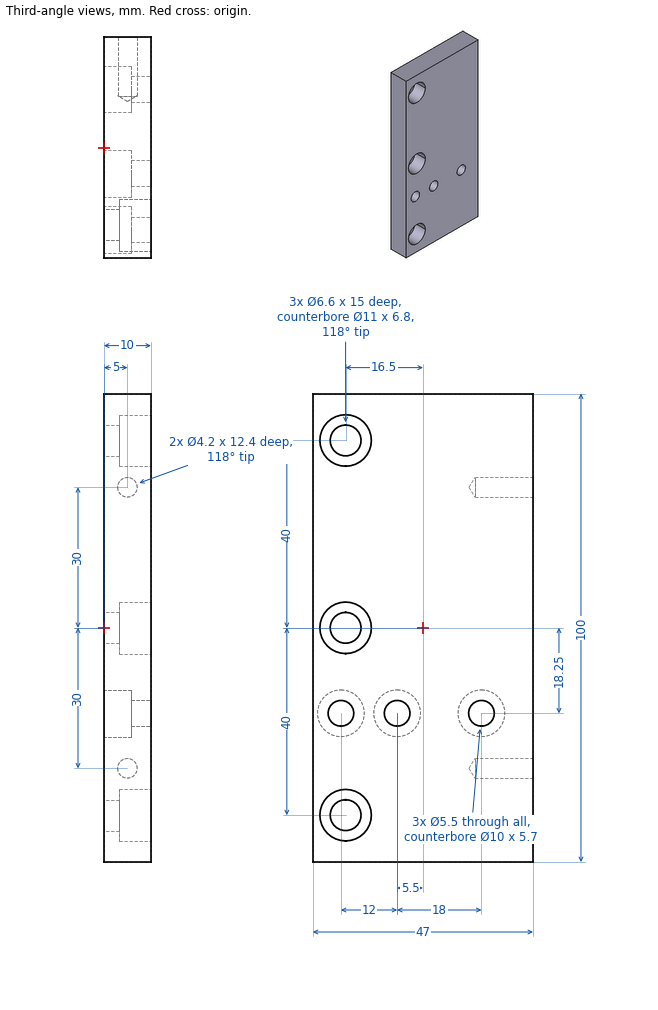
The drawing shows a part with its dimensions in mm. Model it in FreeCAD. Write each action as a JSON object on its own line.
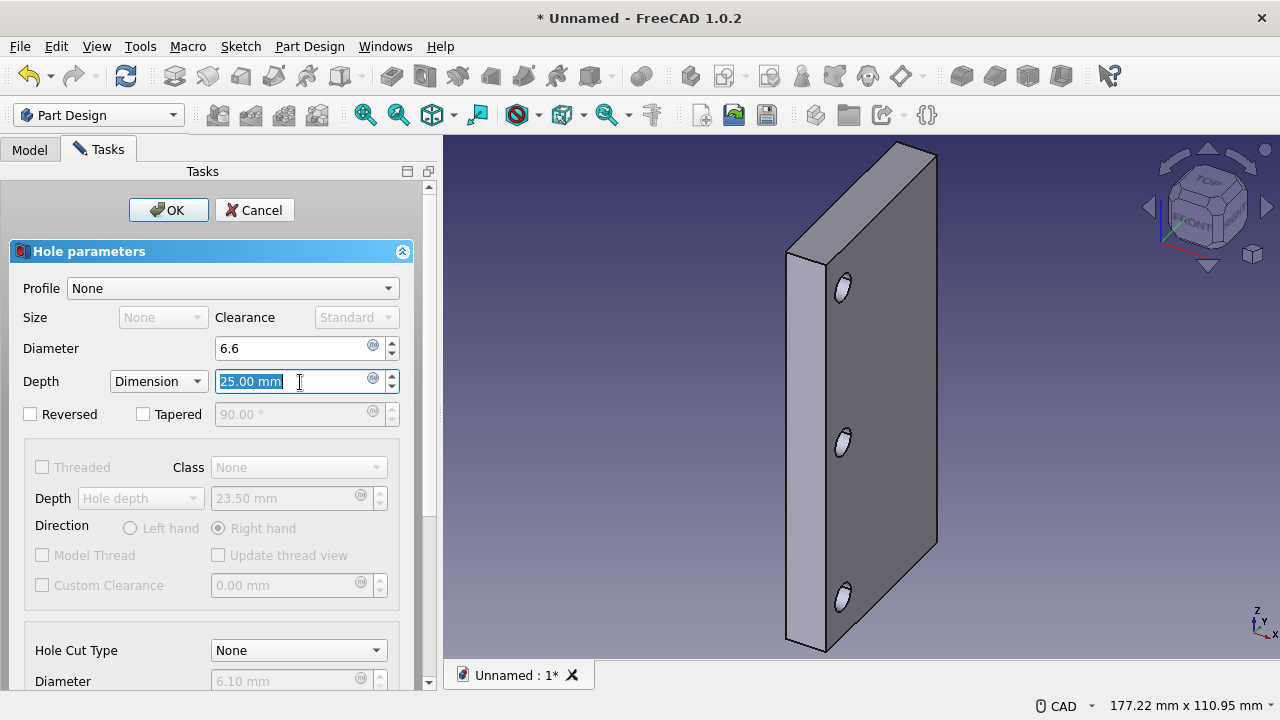
{"action": "type", "text": "15"}
{"action": "key", "text": "Tab"}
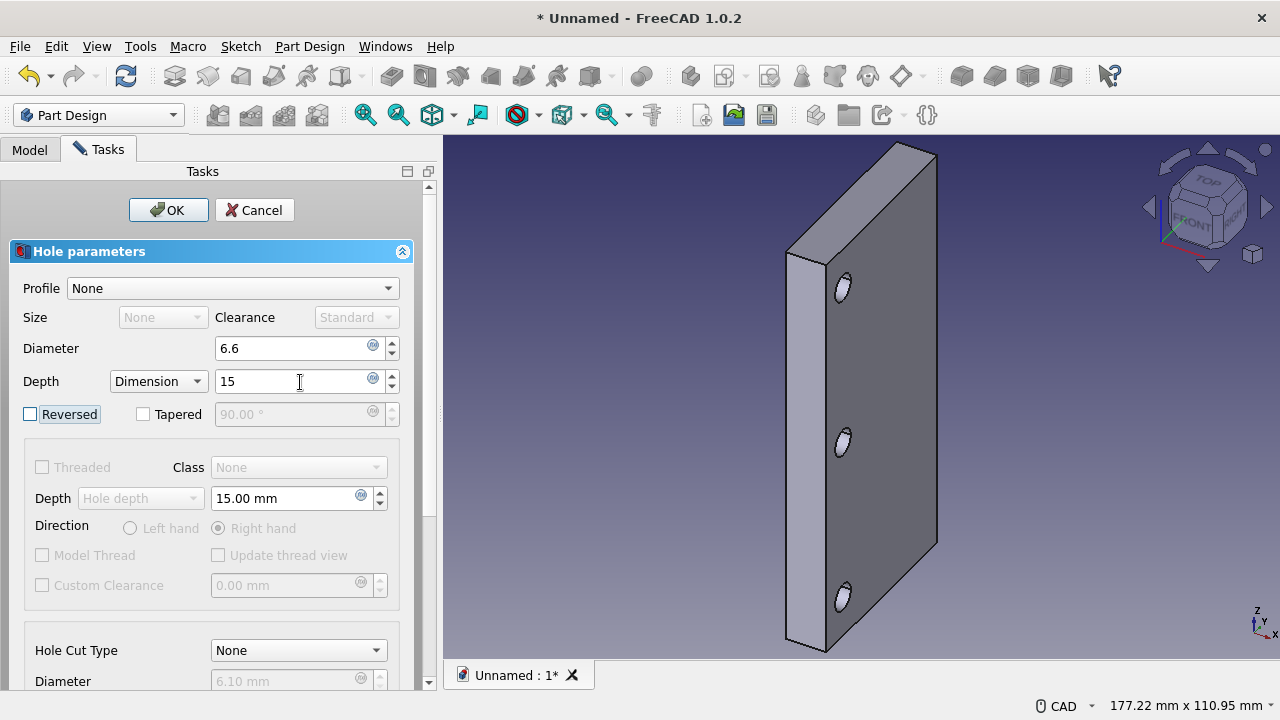
{"action": "left_click", "coordinate": [300, 650]}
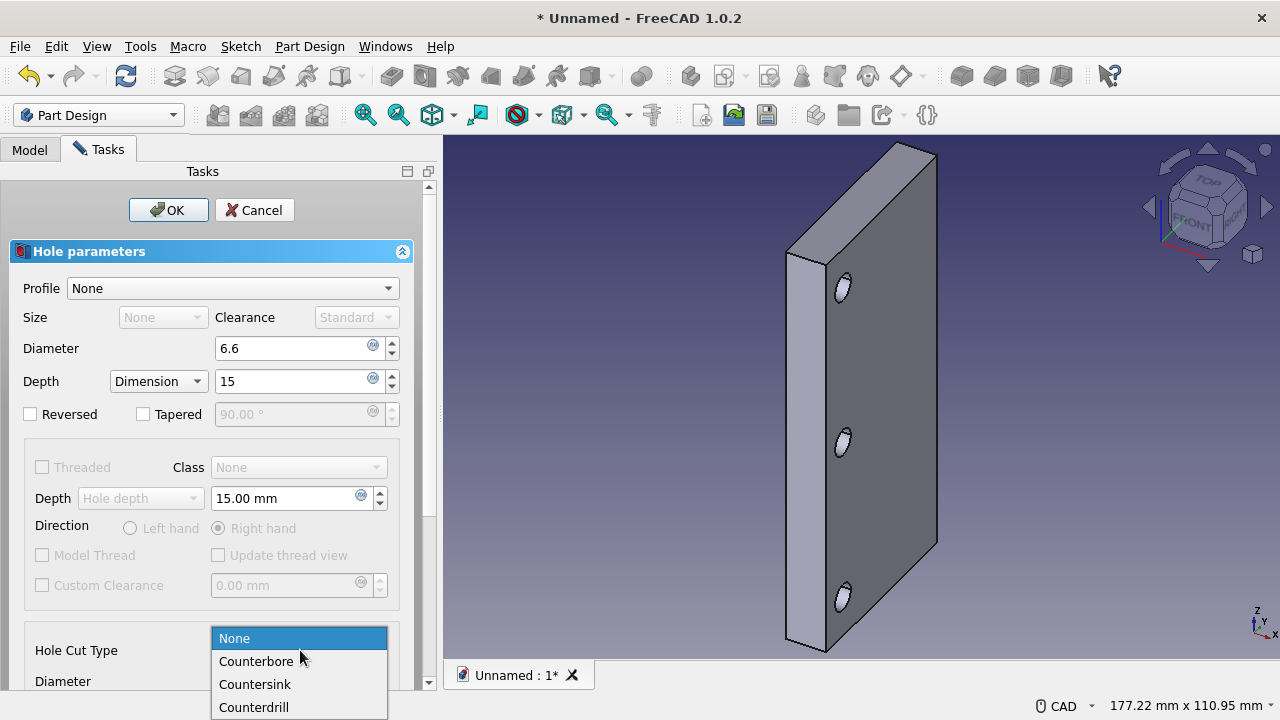
{"action": "left_click", "coordinate": [298, 662]}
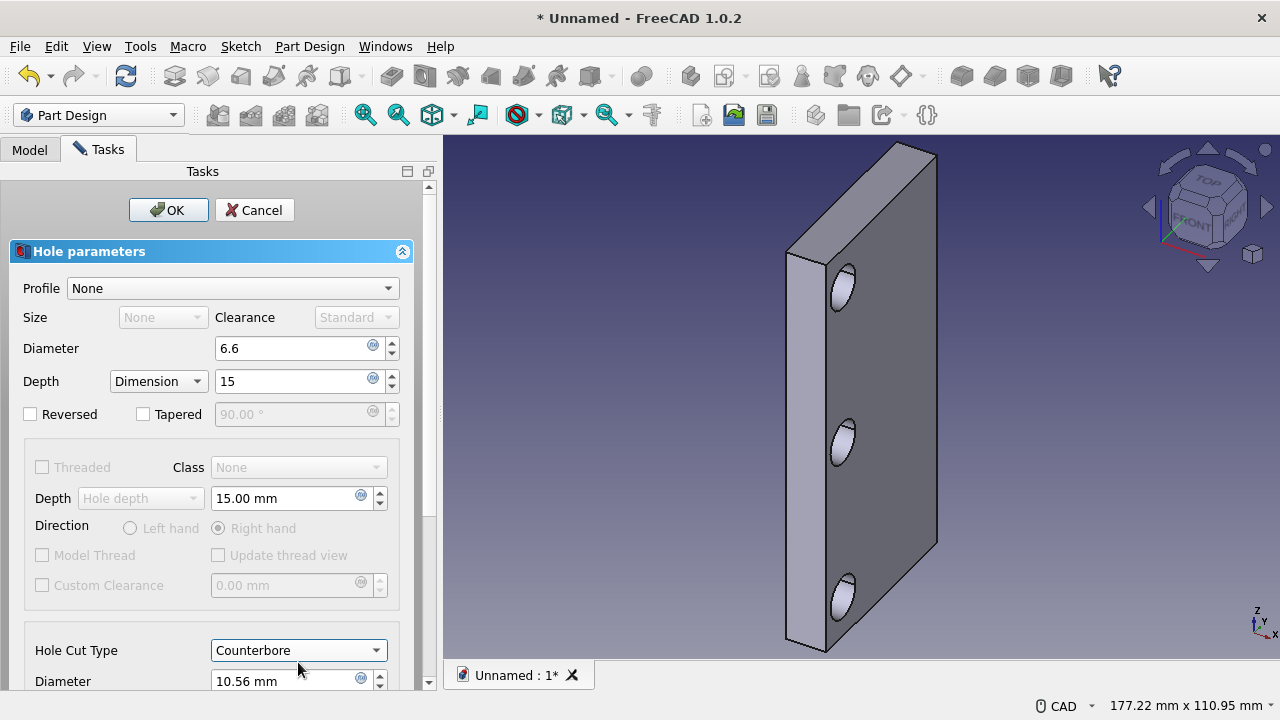
{"action": "scroll", "coordinate": [429, 436], "scroll_direction": "down", "scroll_amount": 2}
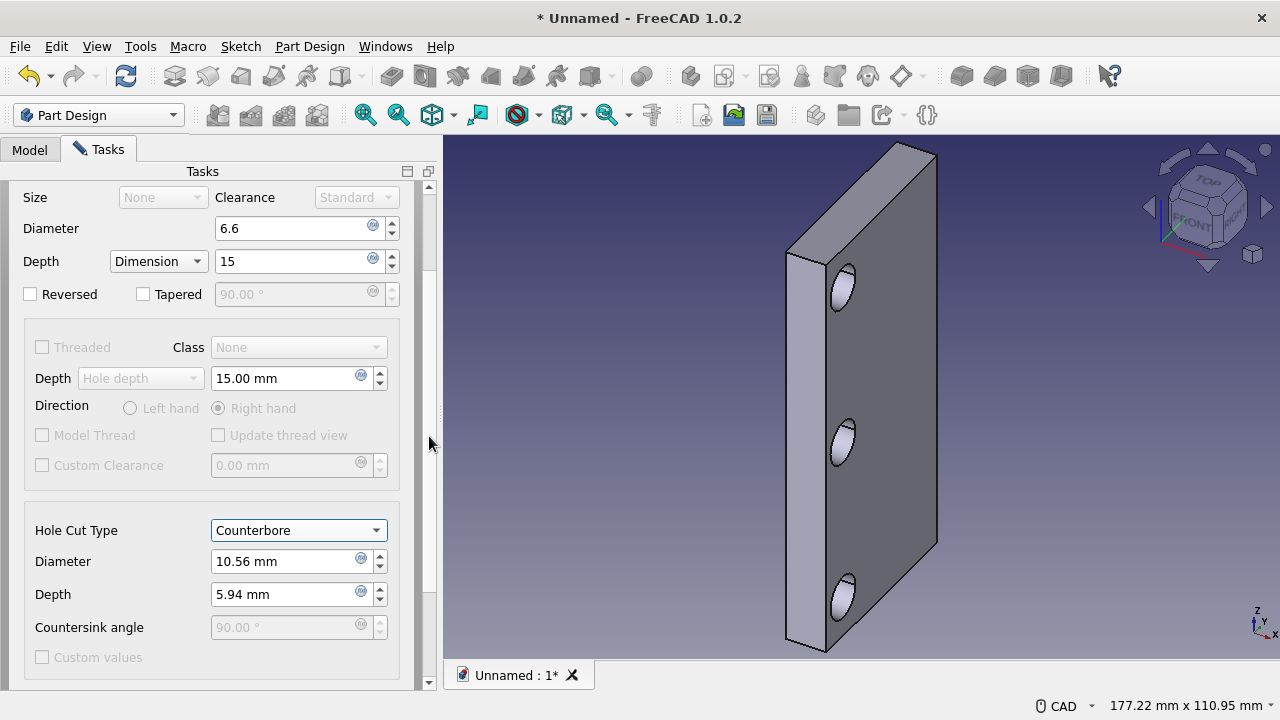
{"action": "triple_click", "coordinate": [292, 562]}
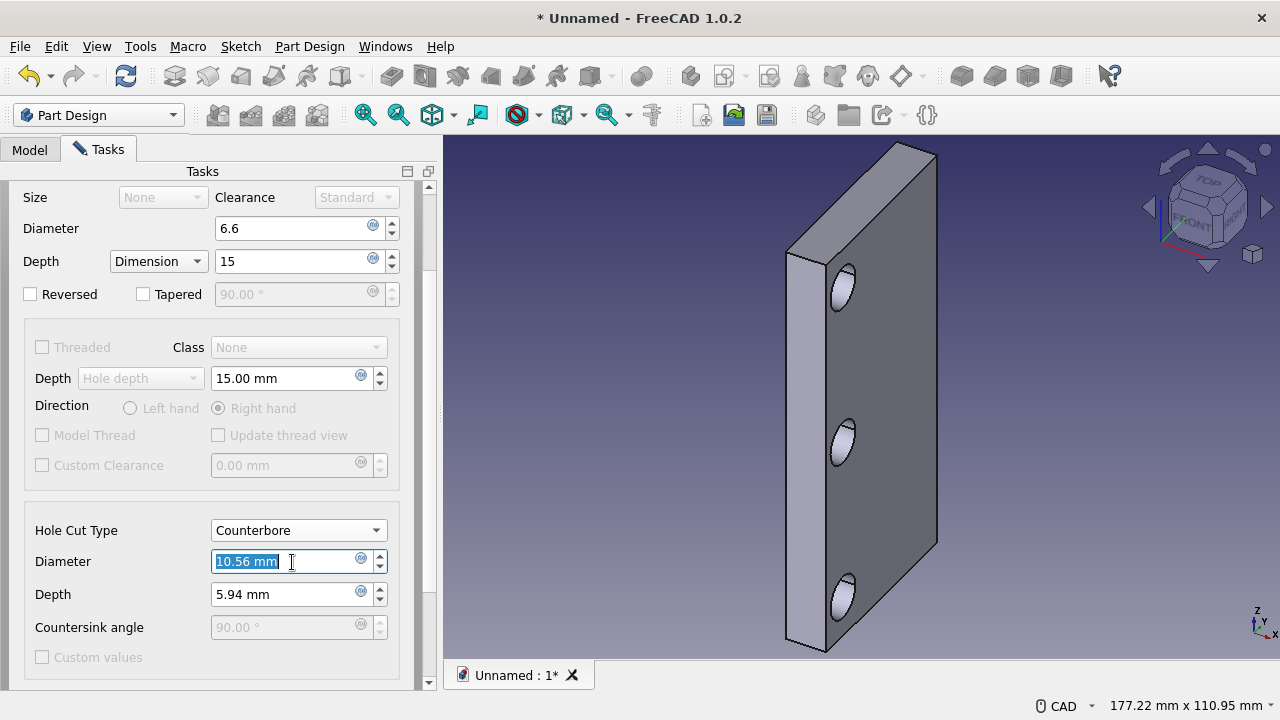
{"action": "type", "text": "11"}
{"action": "key", "text": "Tab"}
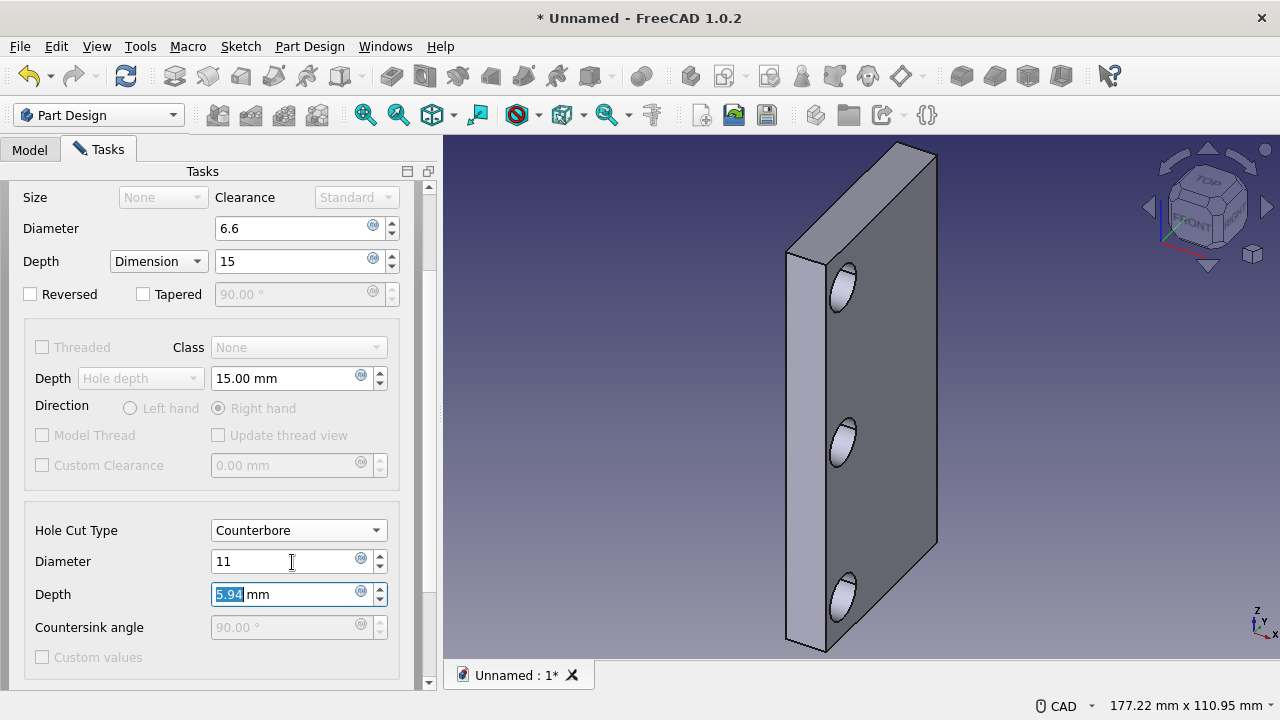
{"action": "type", "text": "6.8"}
{"action": "key", "text": "Tab"}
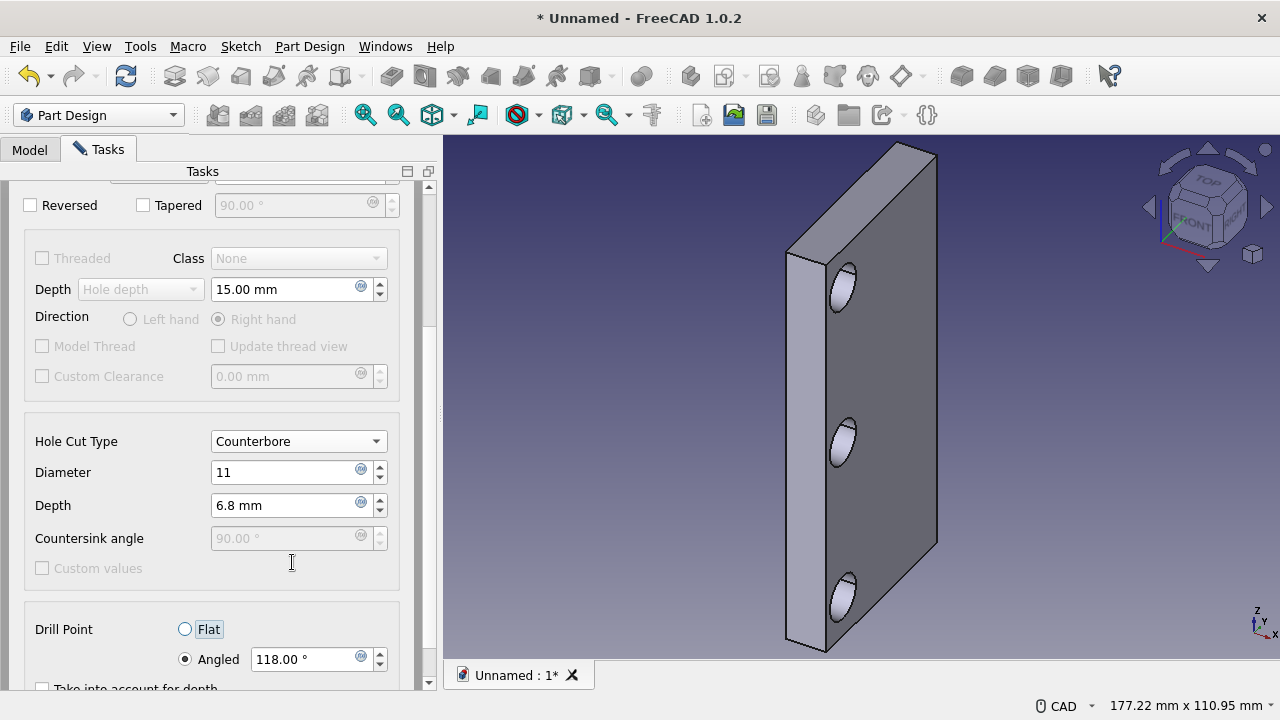
{"action": "scroll", "coordinate": [429, 436], "scroll_direction": "up", "scroll_amount": 5}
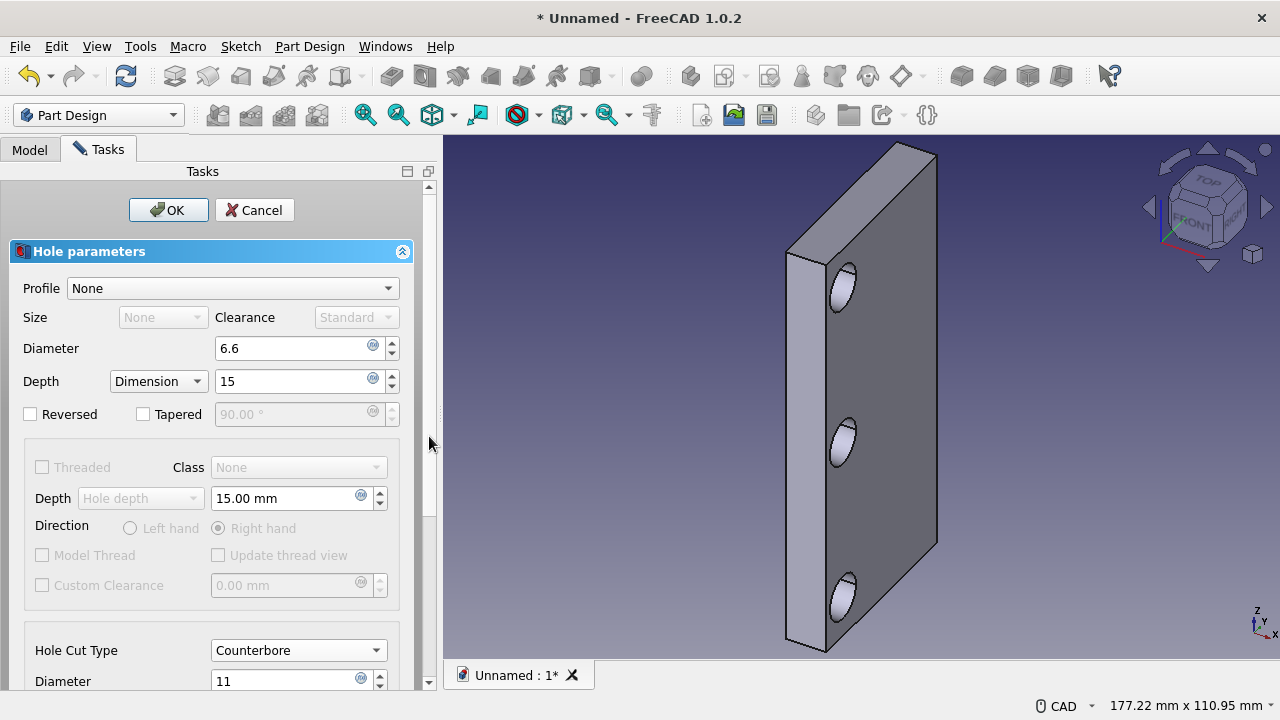
{"action": "left_click", "coordinate": [169, 210]}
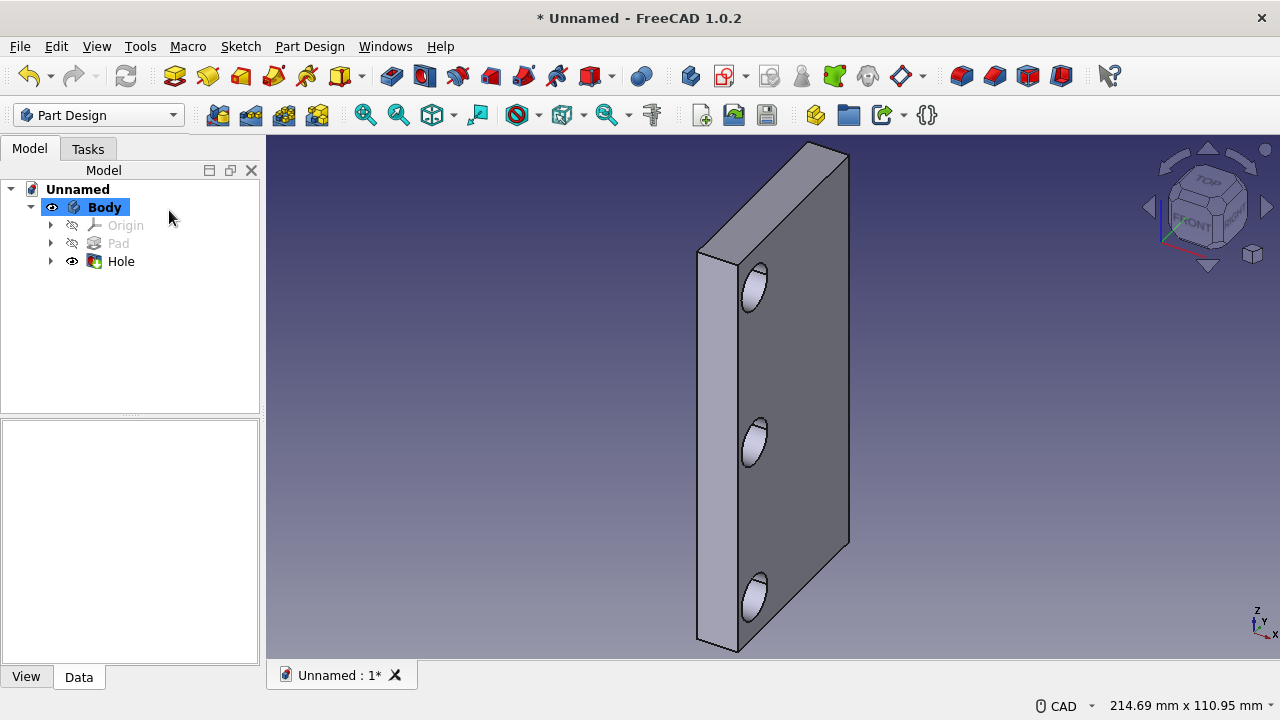
{"action": "key", "text": "6"}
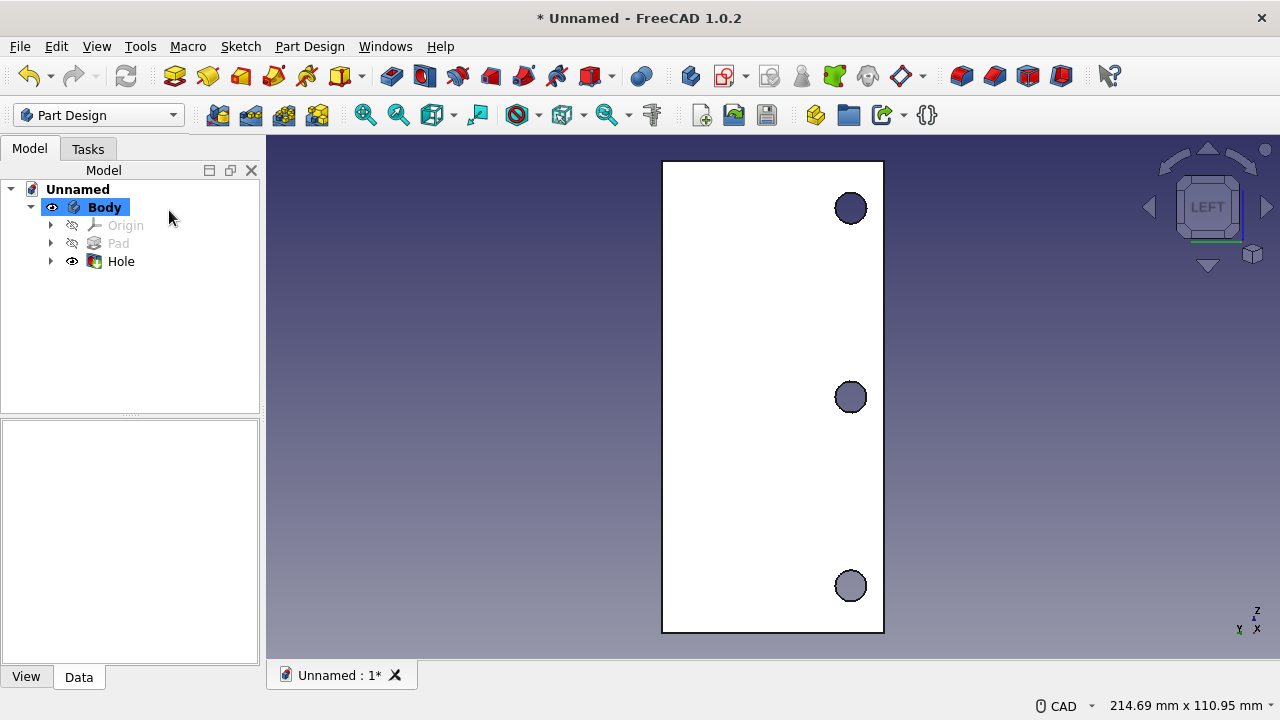
{"action": "left_click", "coordinate": [773, 329]}